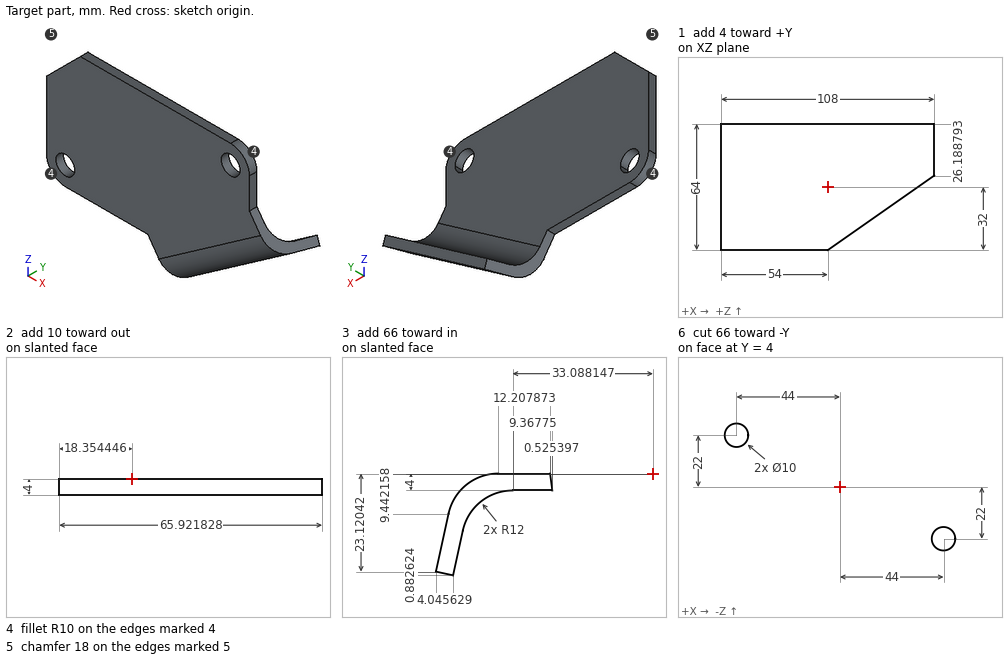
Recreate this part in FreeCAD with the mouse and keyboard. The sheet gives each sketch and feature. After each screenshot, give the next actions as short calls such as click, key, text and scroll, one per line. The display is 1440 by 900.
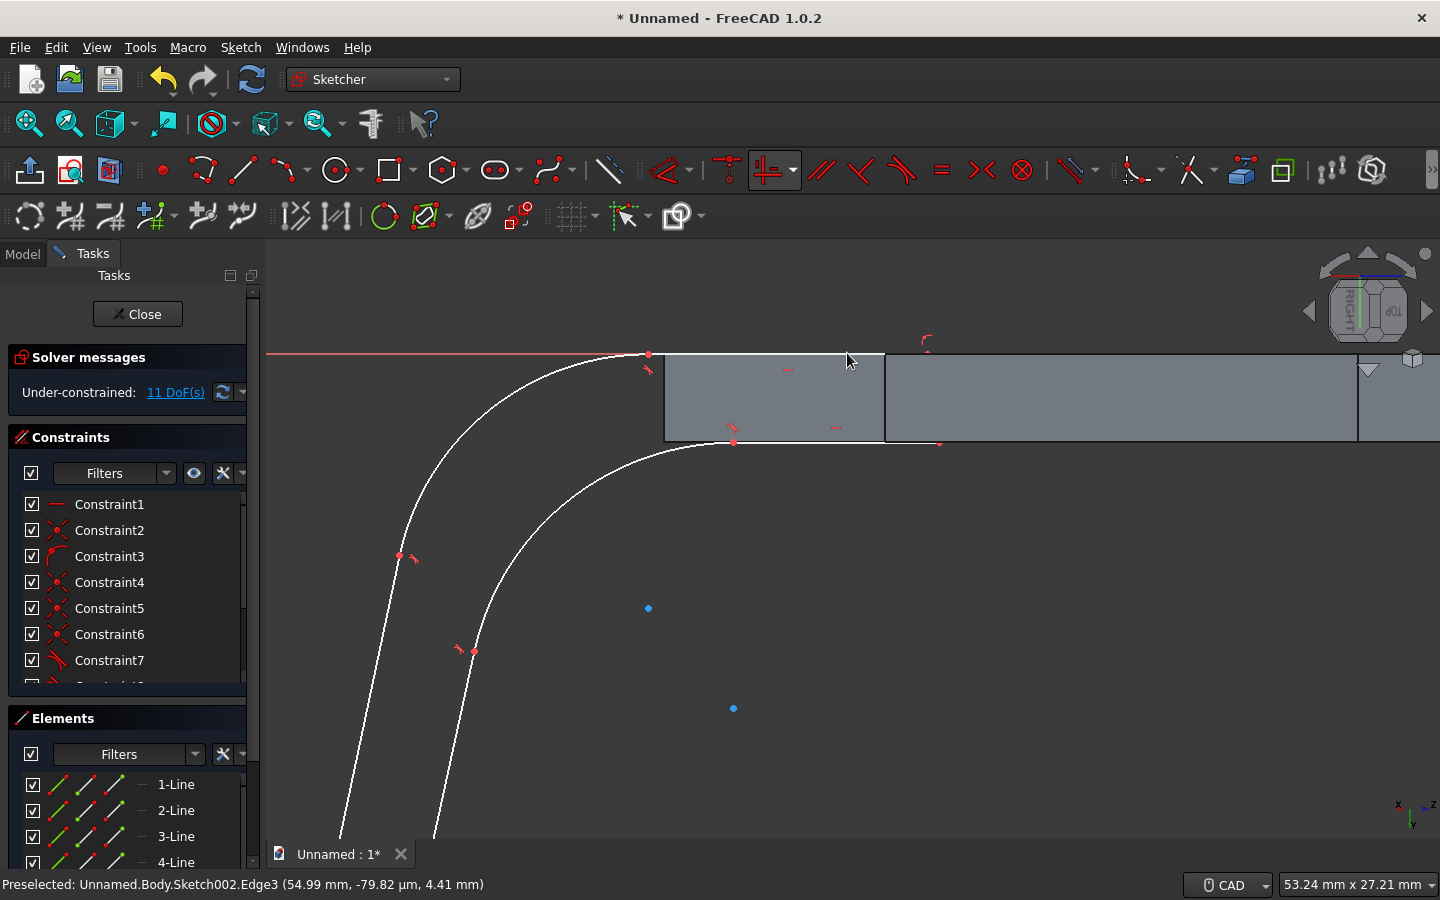
click(547, 375)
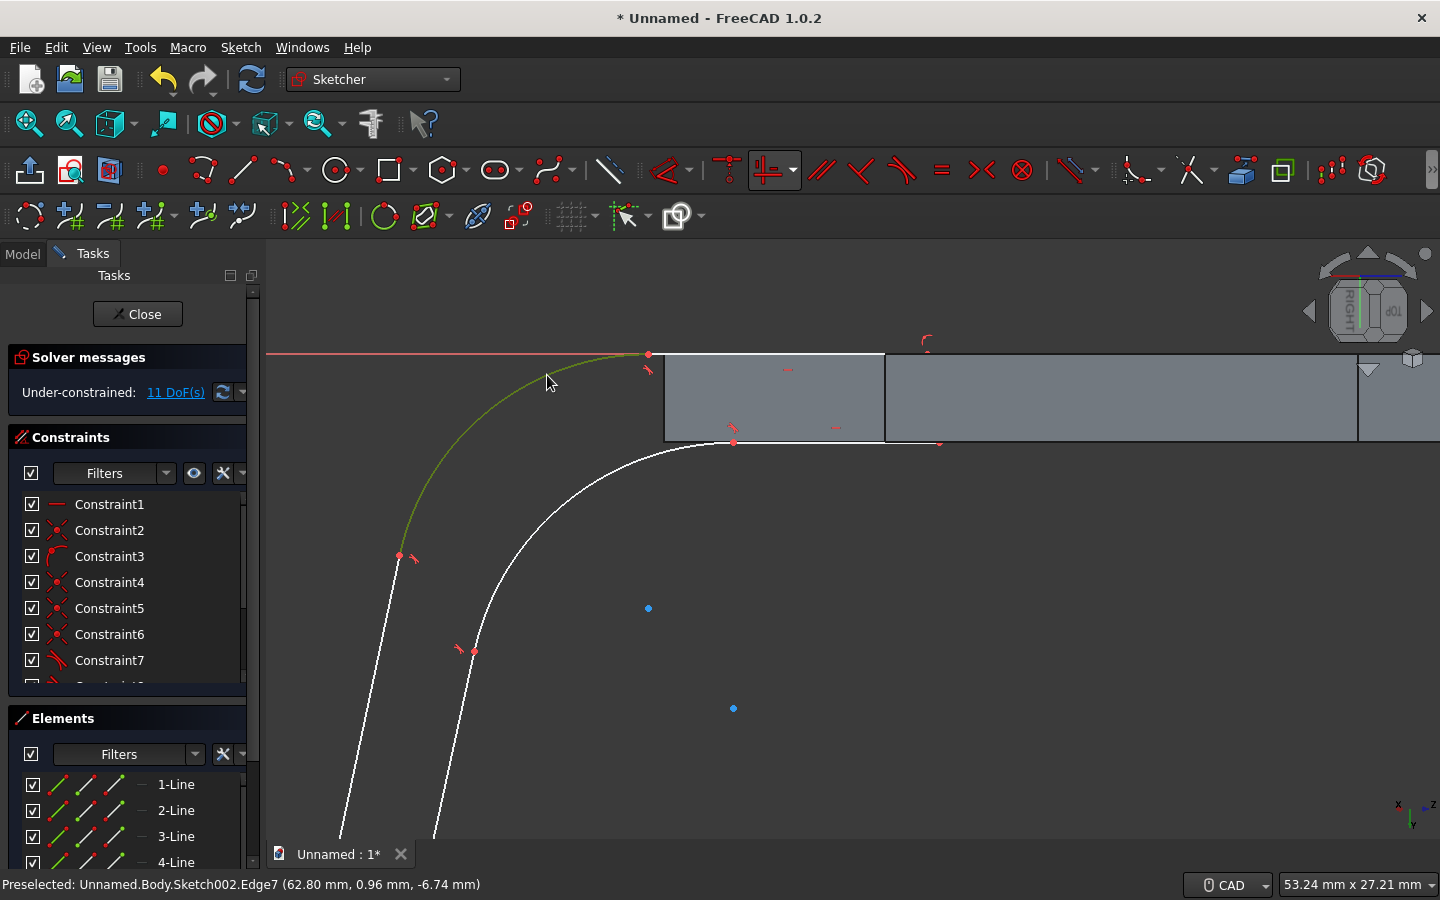
click(629, 464)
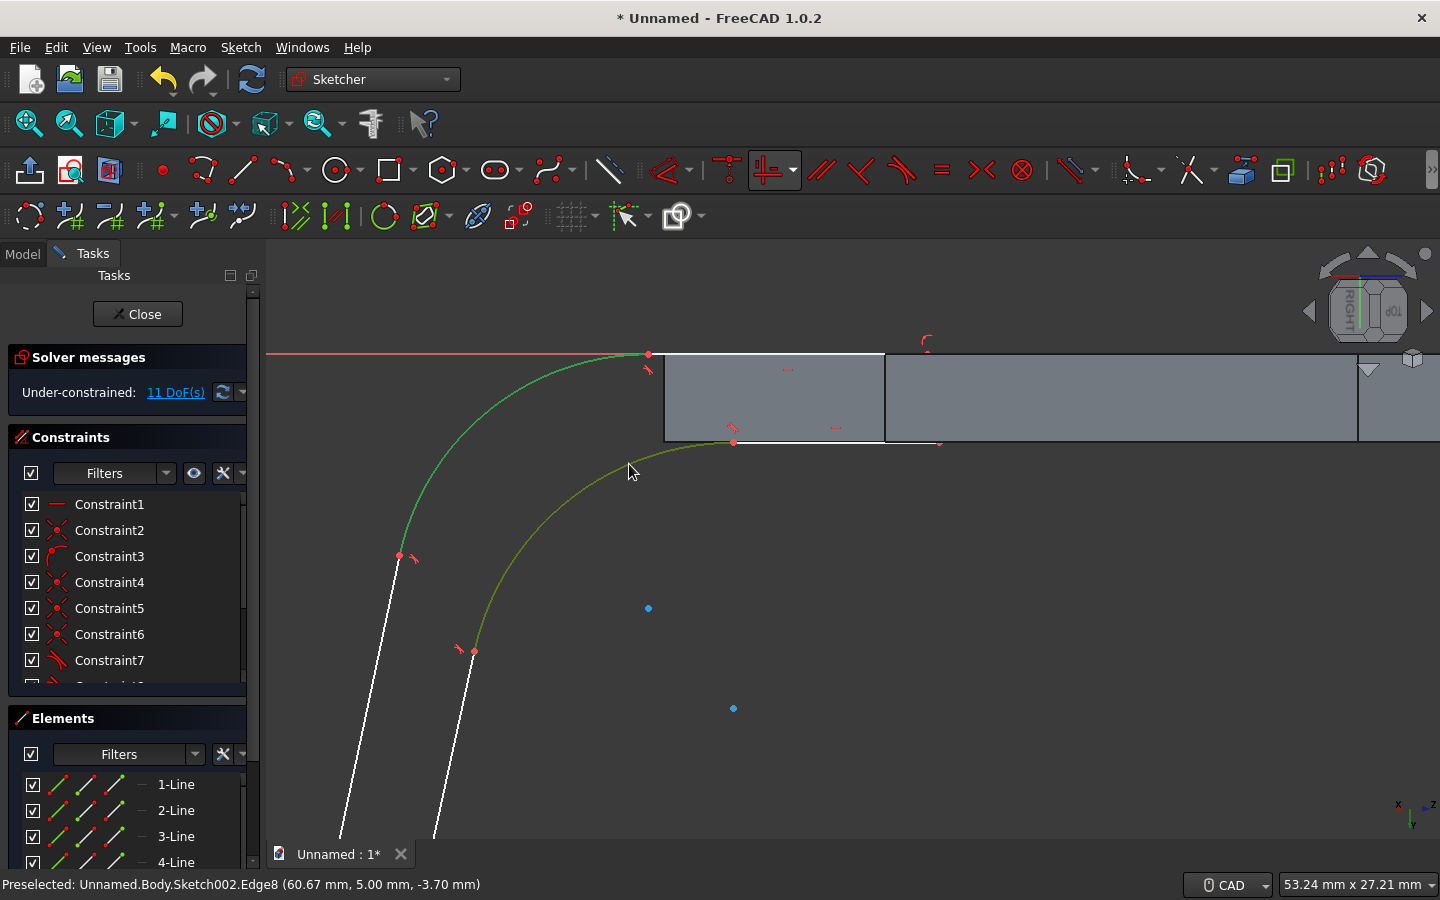
key(e)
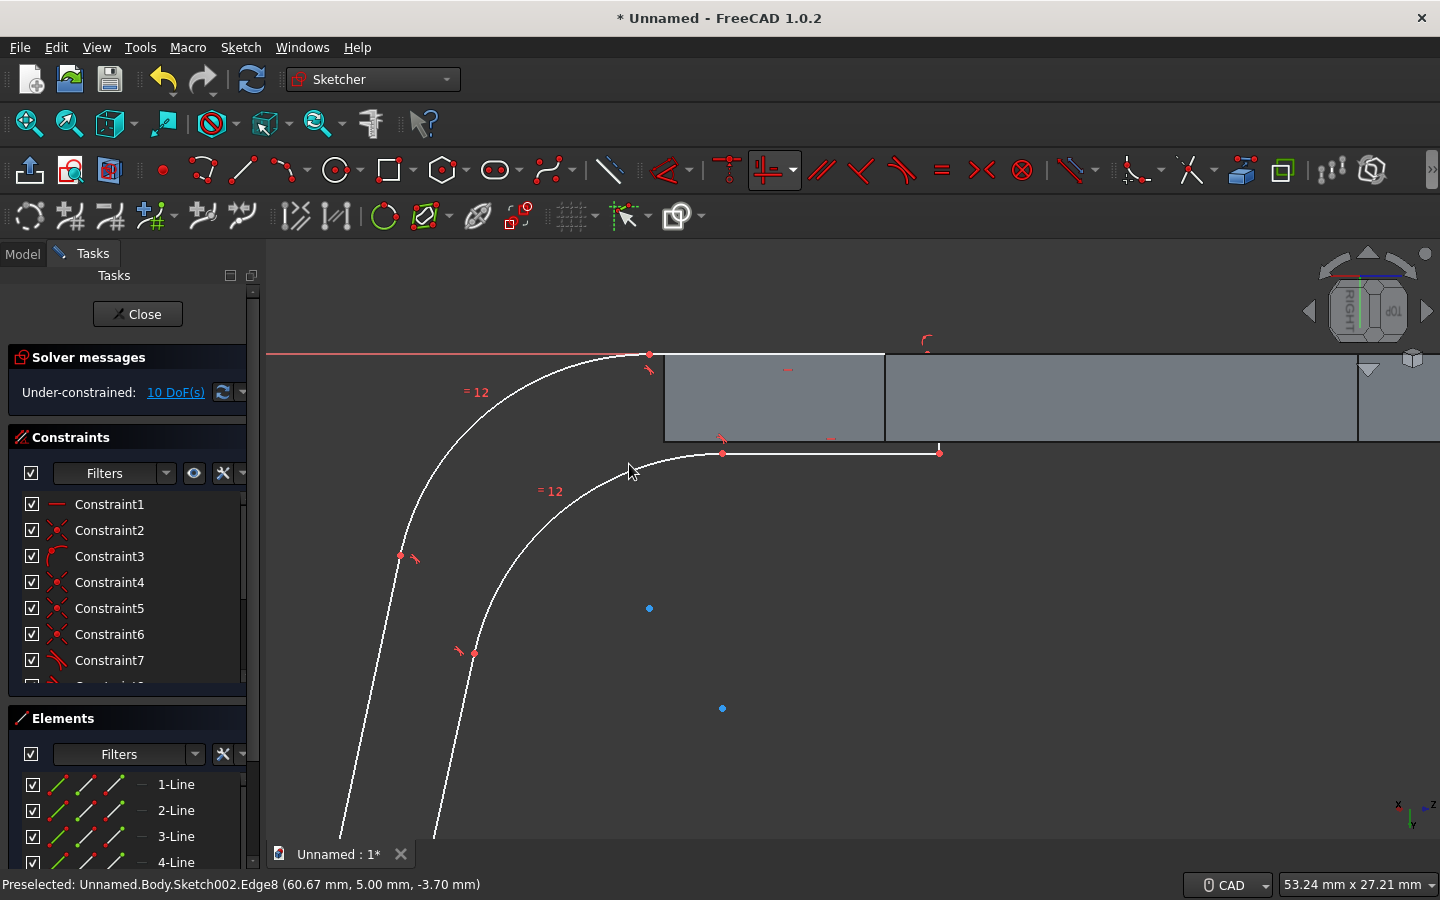
click(548, 375)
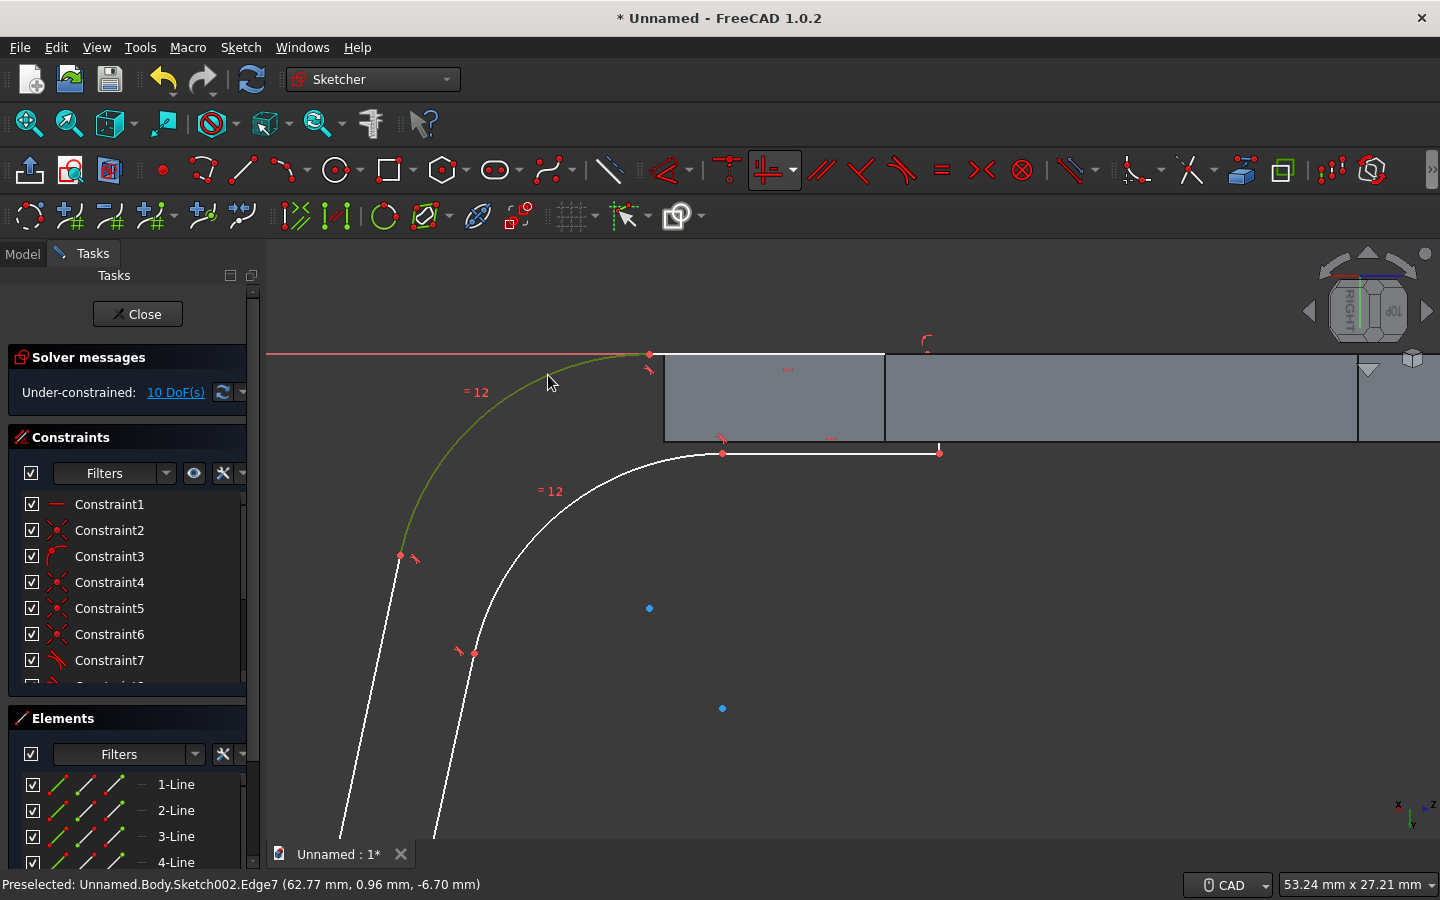
click(692, 170)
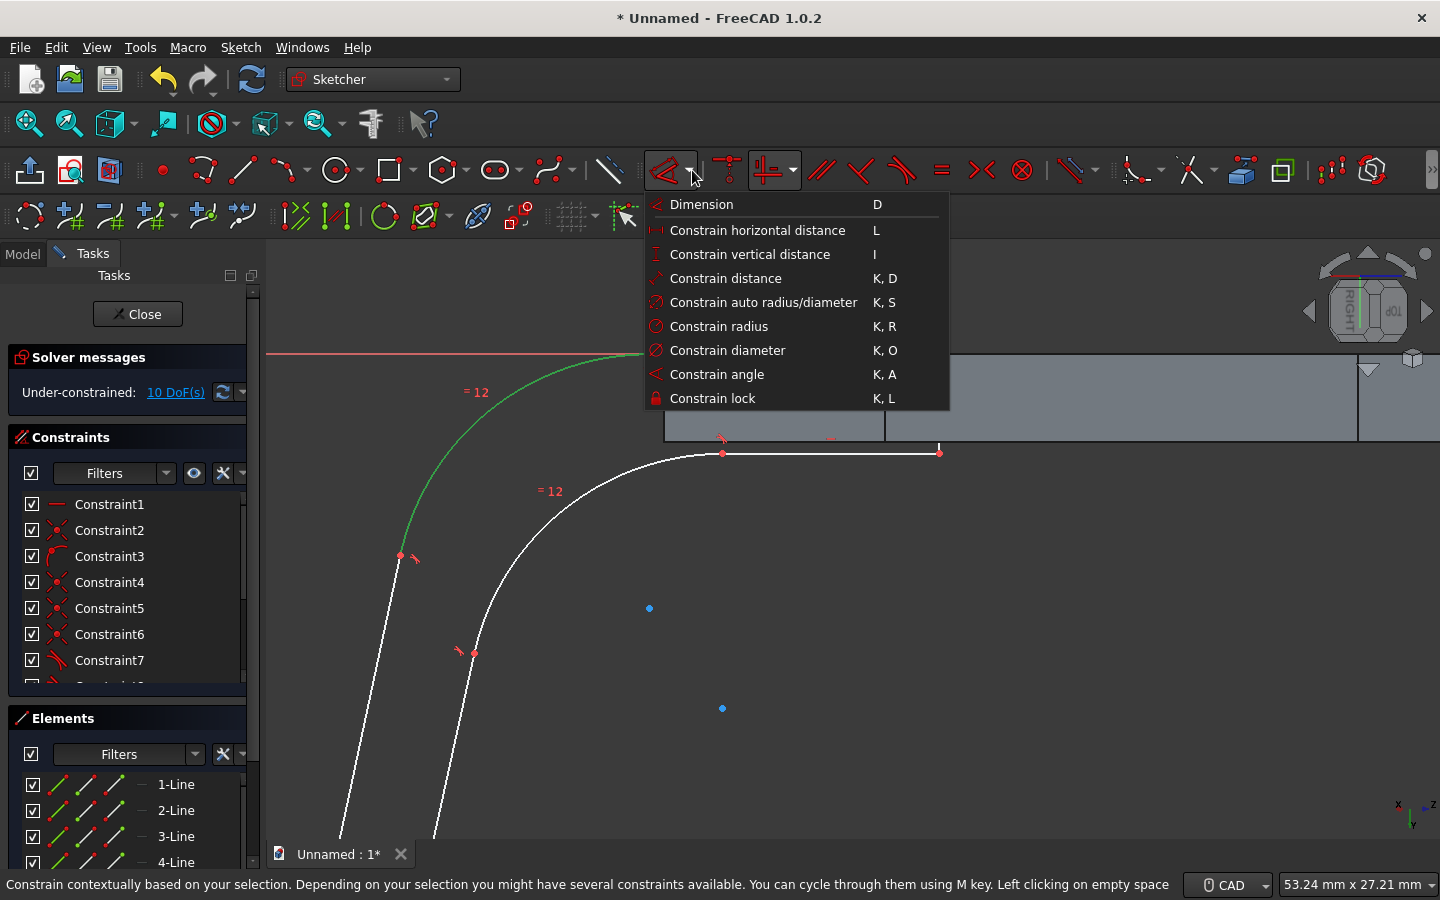
click(797, 326)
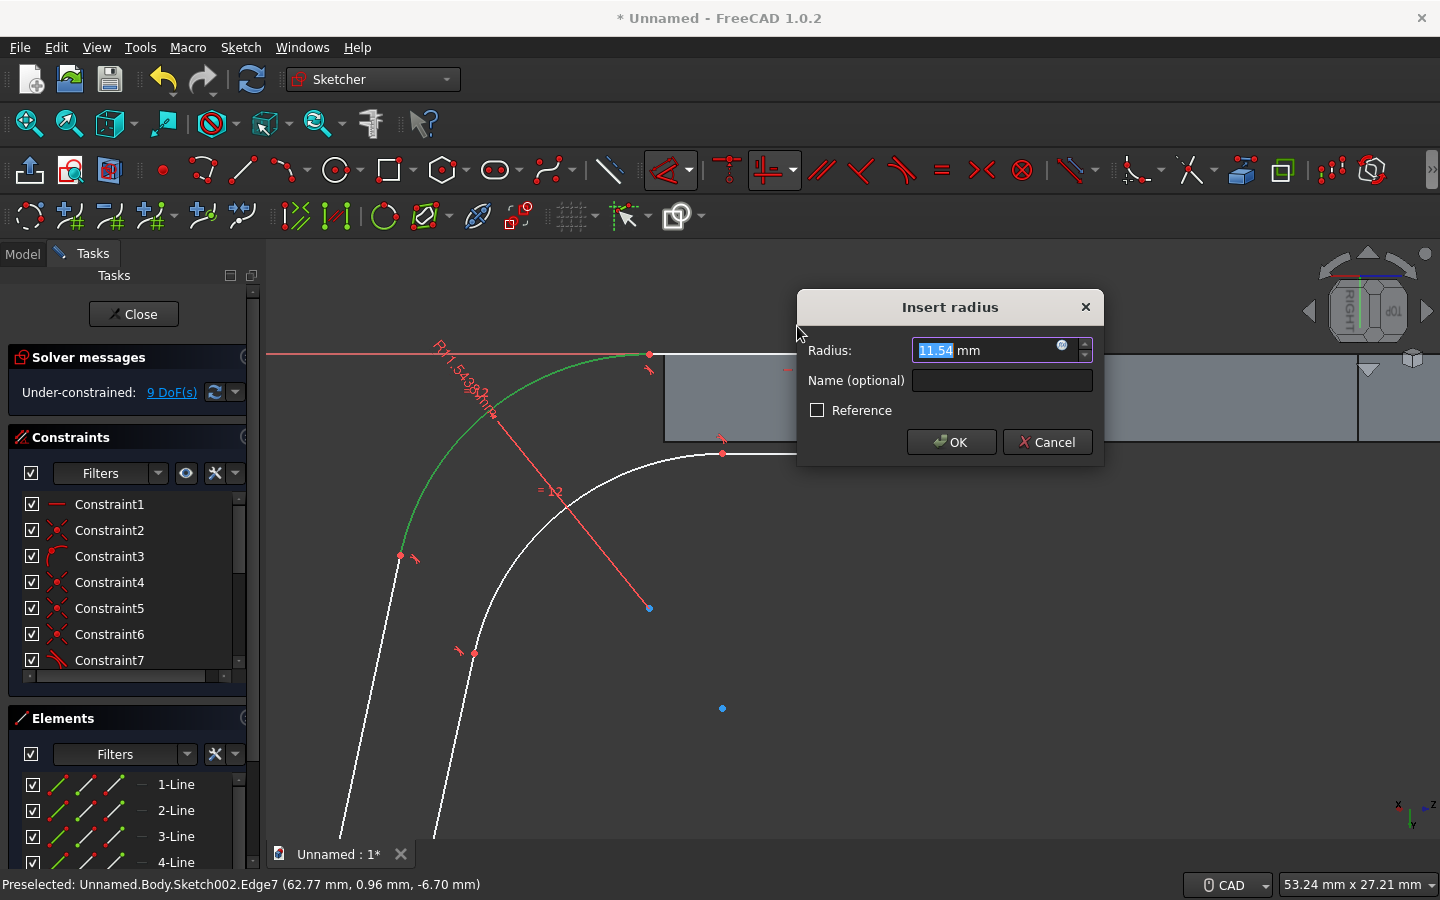
text(12)
key(Return)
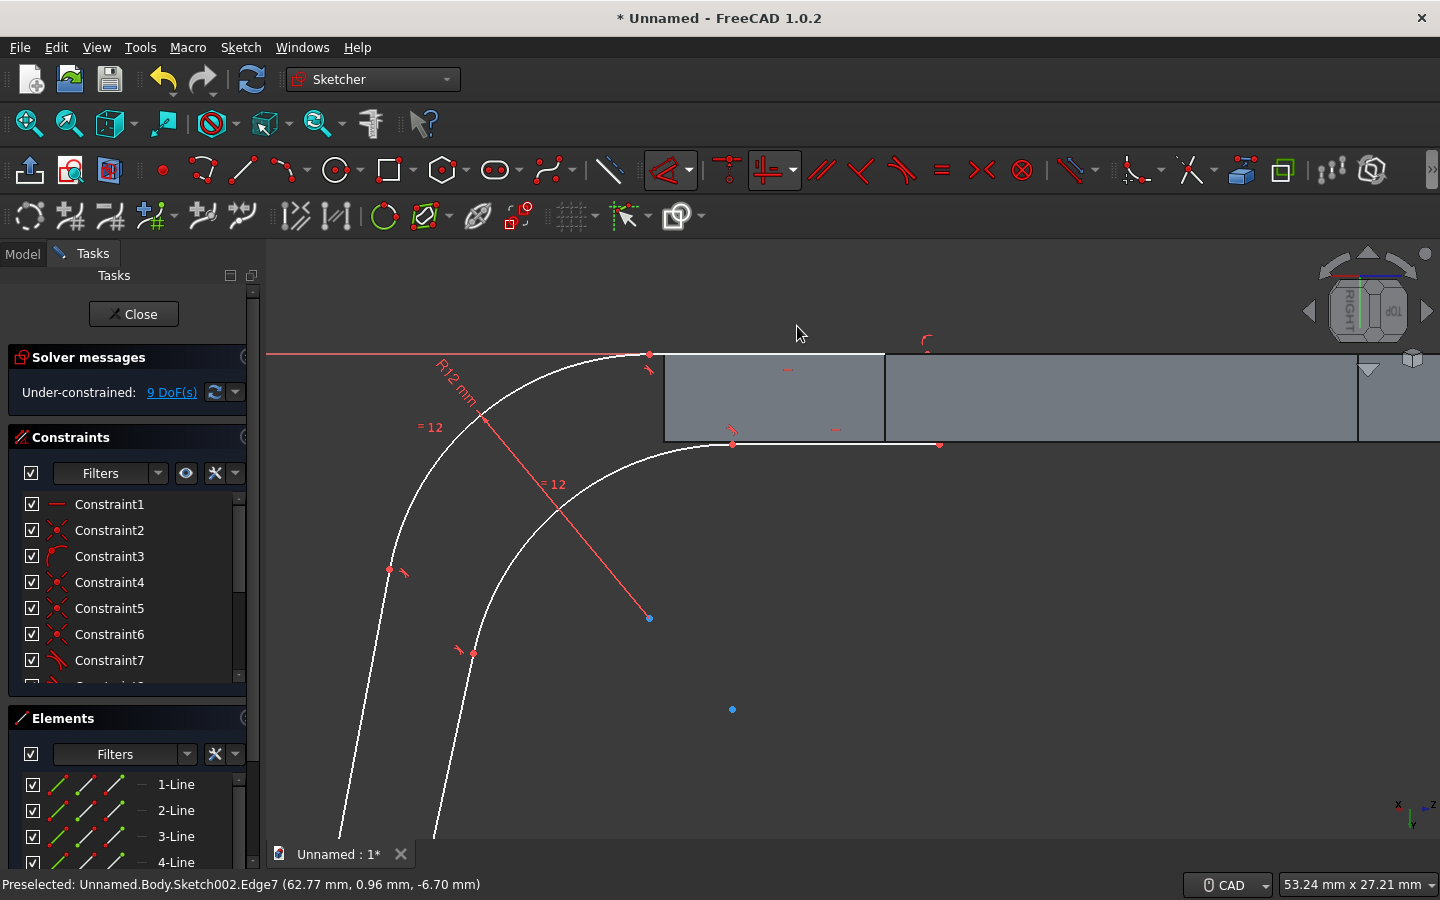
click(732, 444)